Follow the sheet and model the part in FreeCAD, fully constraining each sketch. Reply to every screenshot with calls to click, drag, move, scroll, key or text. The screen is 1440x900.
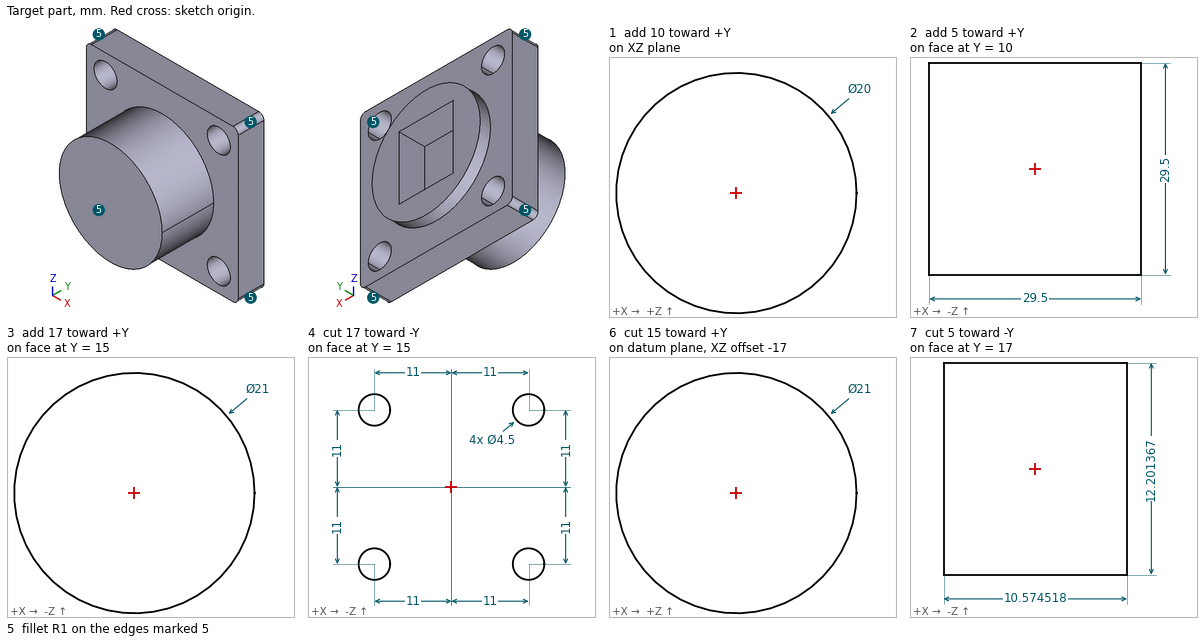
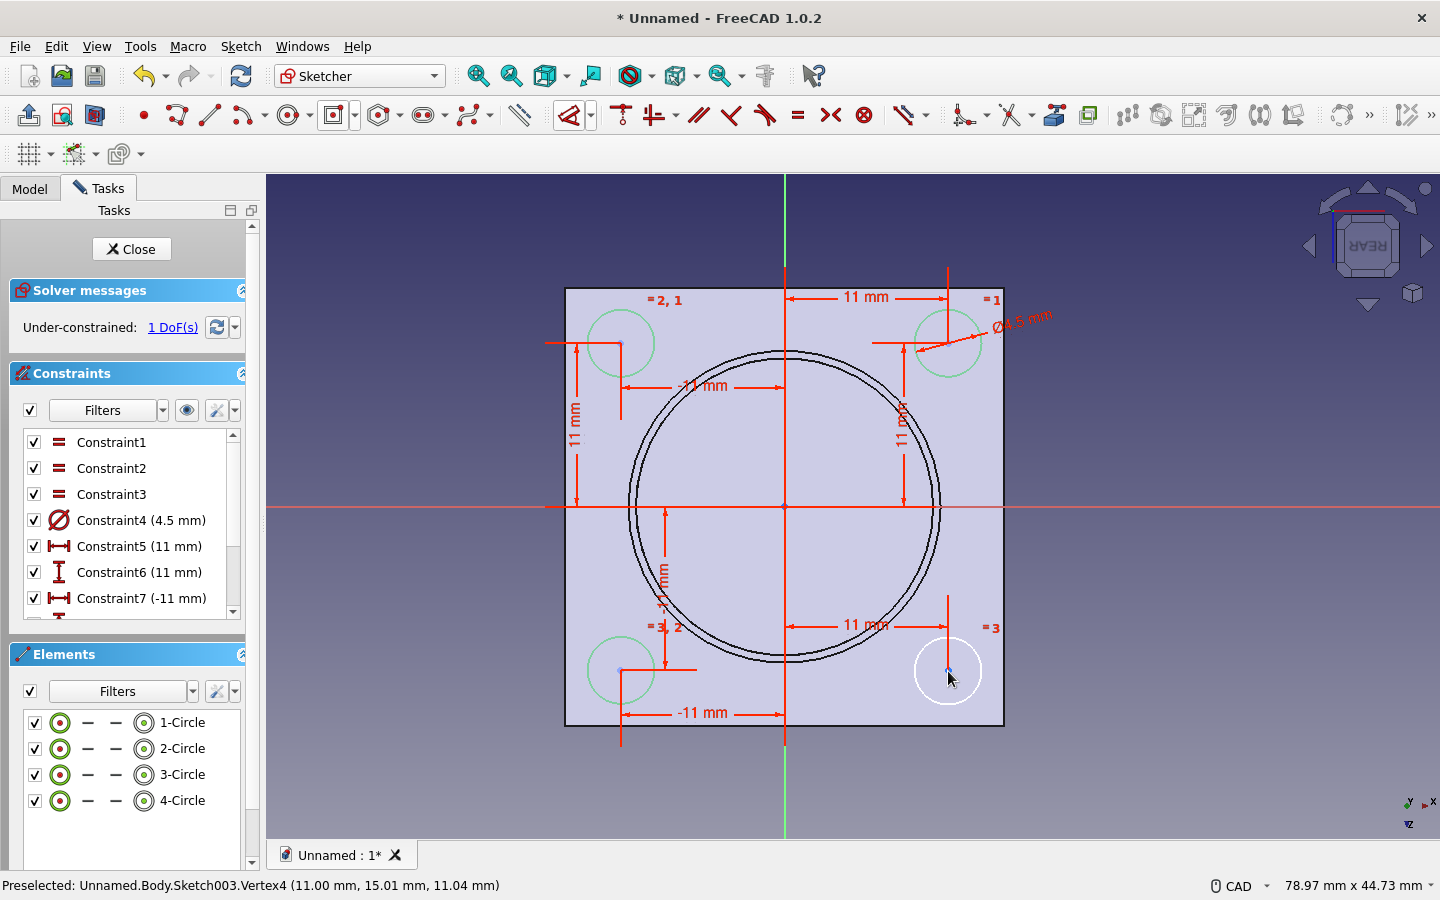
click(948, 671)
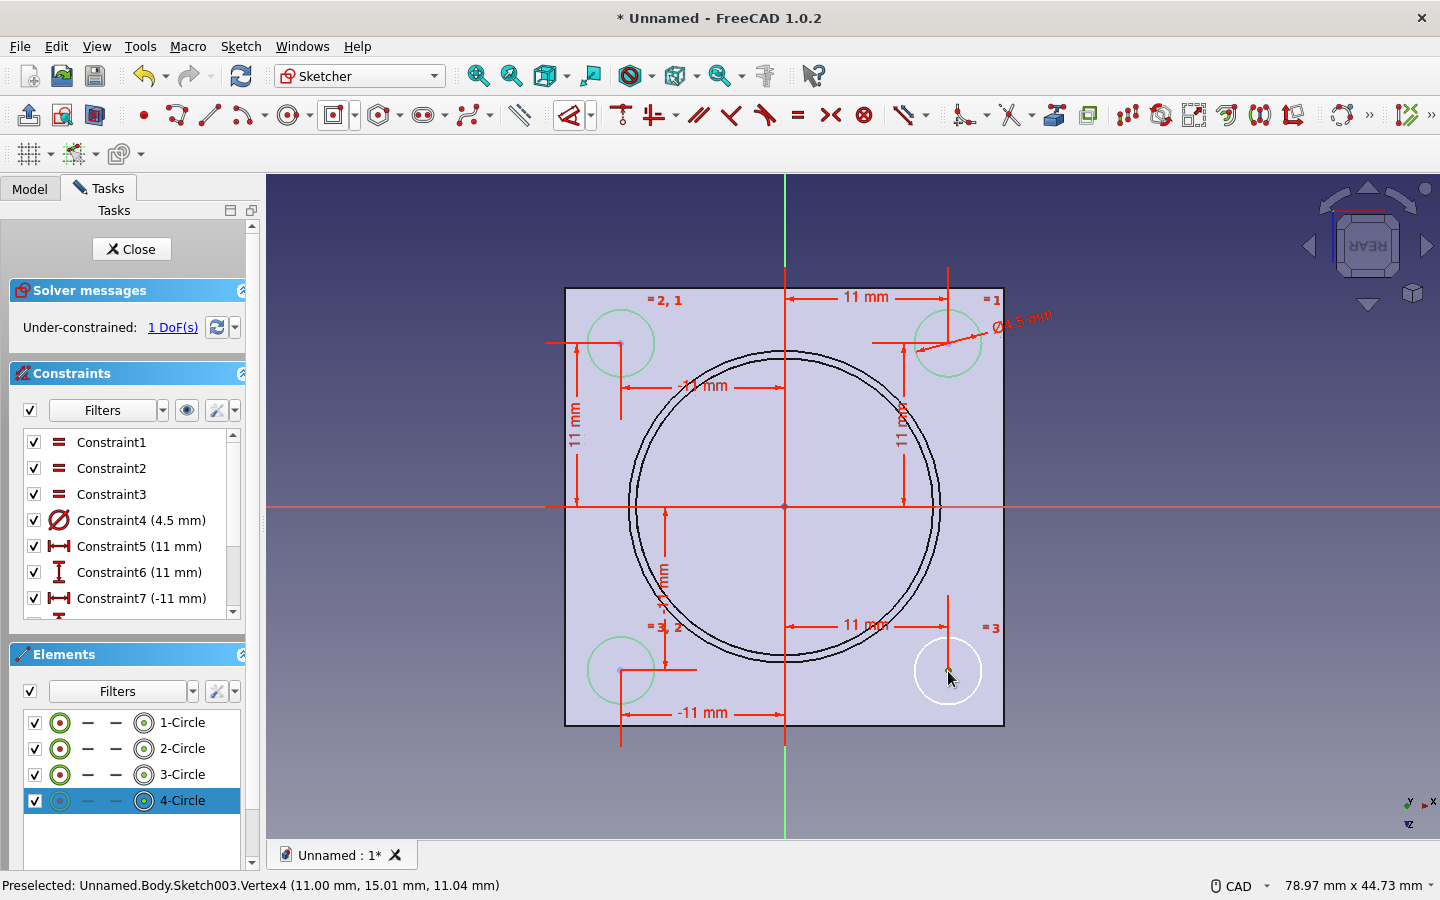
key(i)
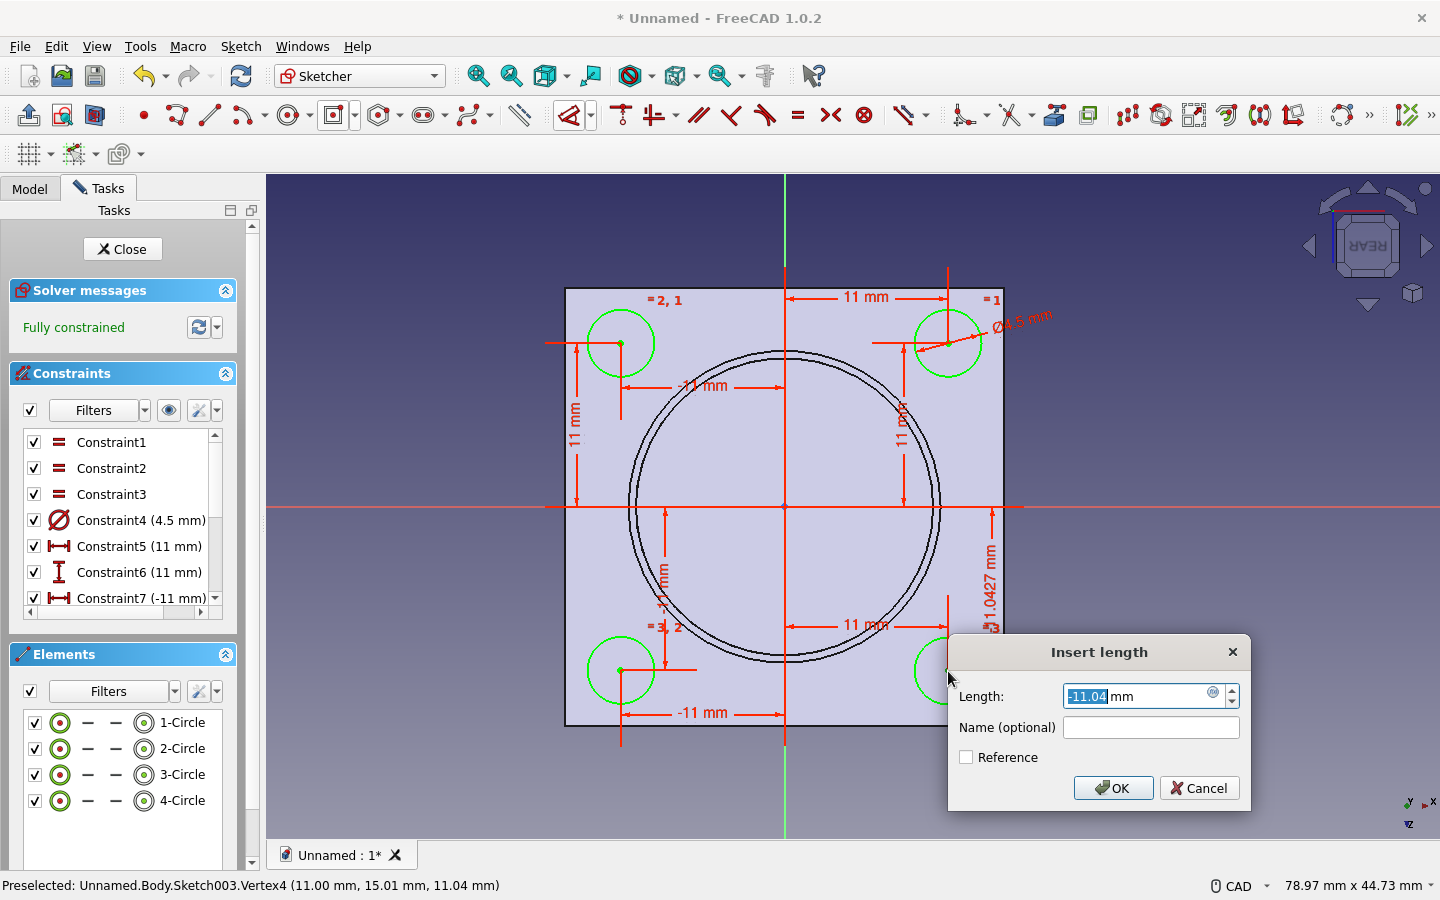
text(-11)
key(Return)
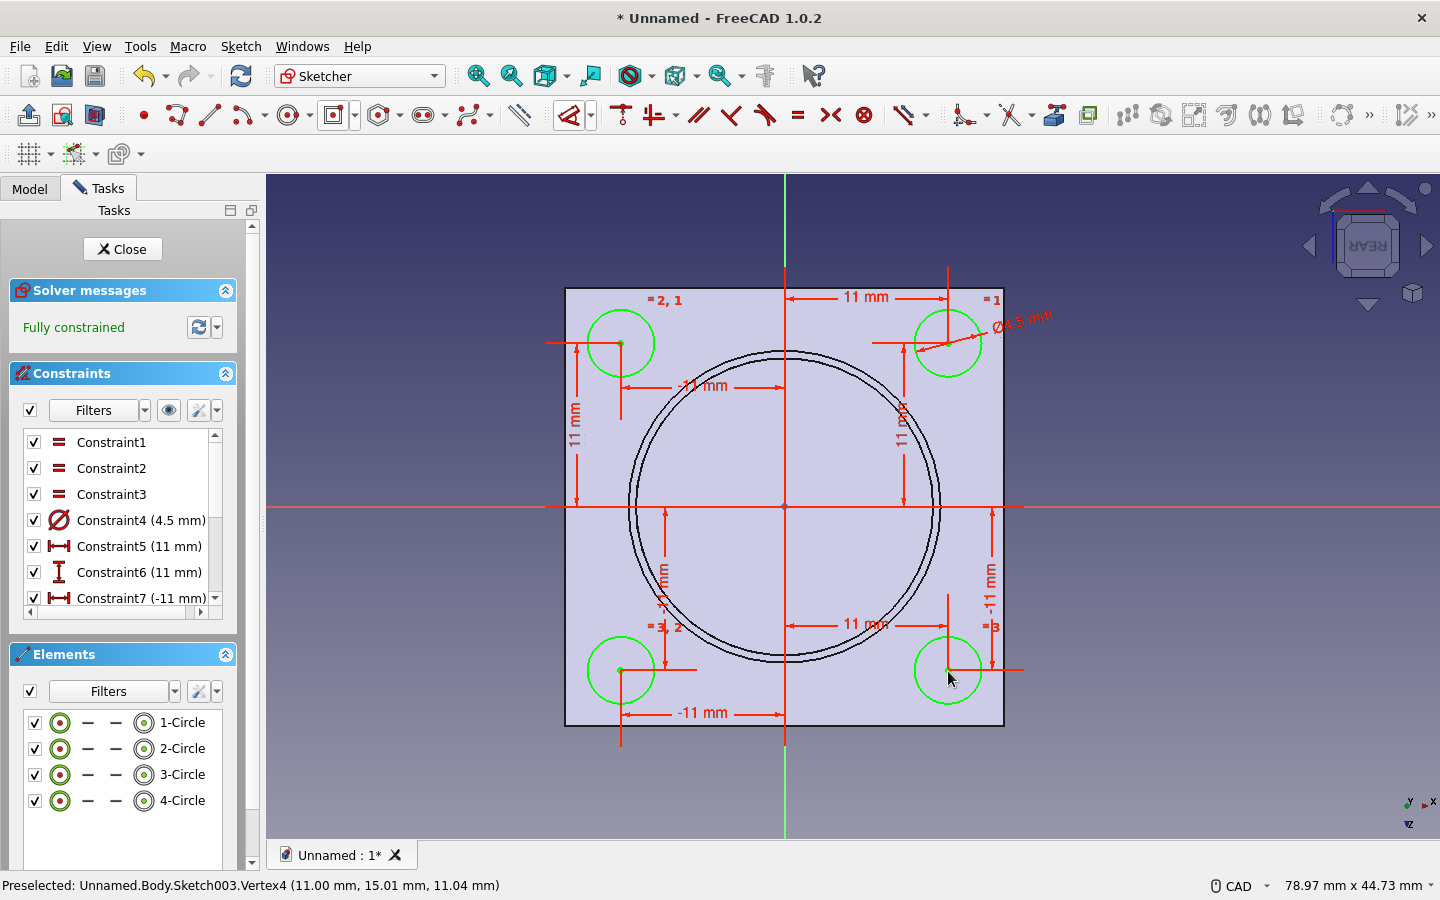
click(123, 249)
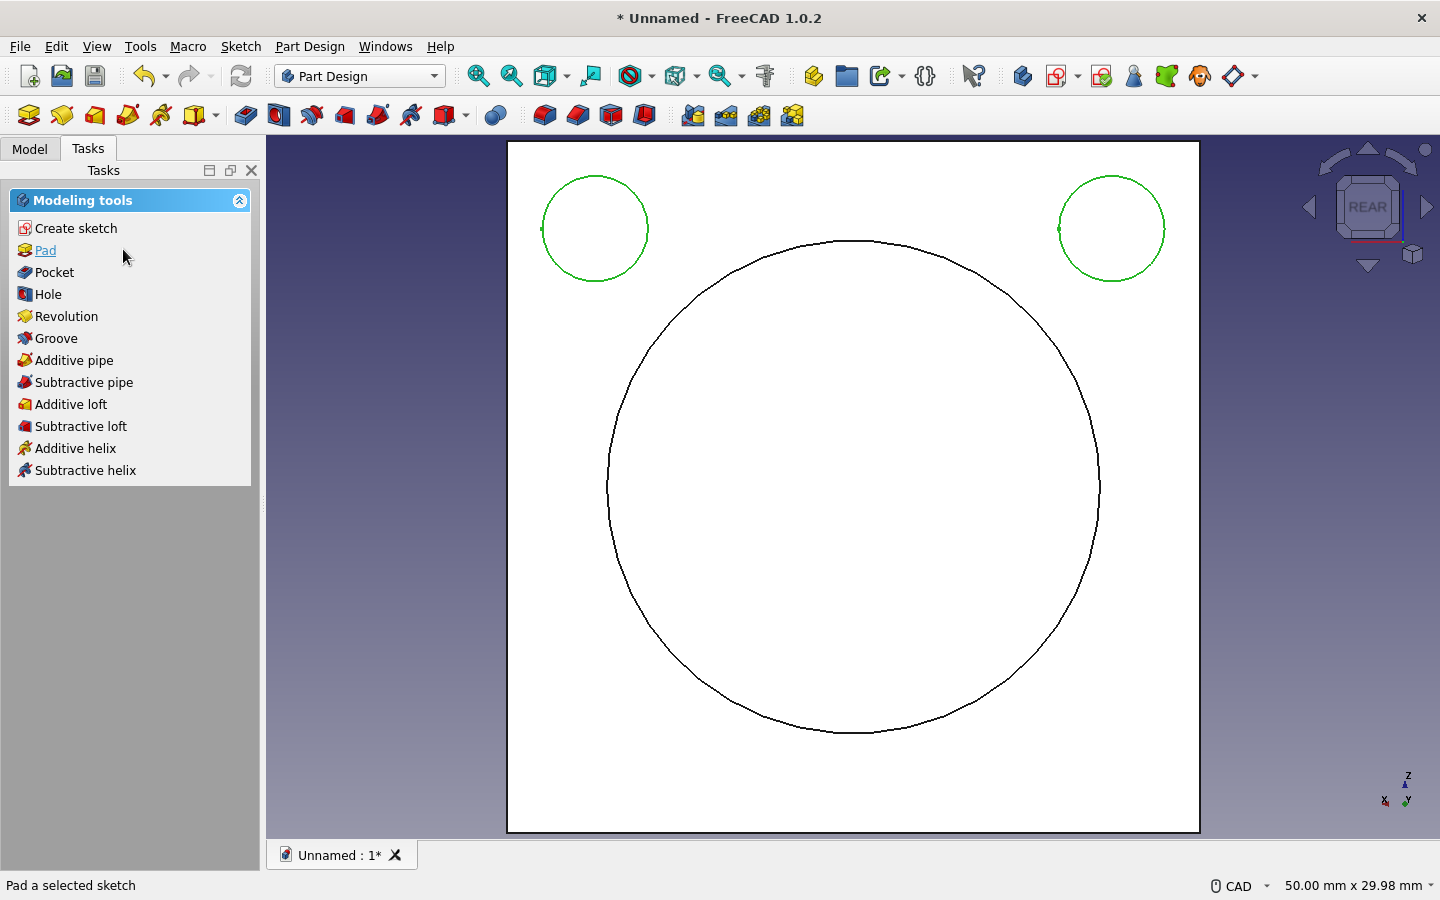
click(246, 116)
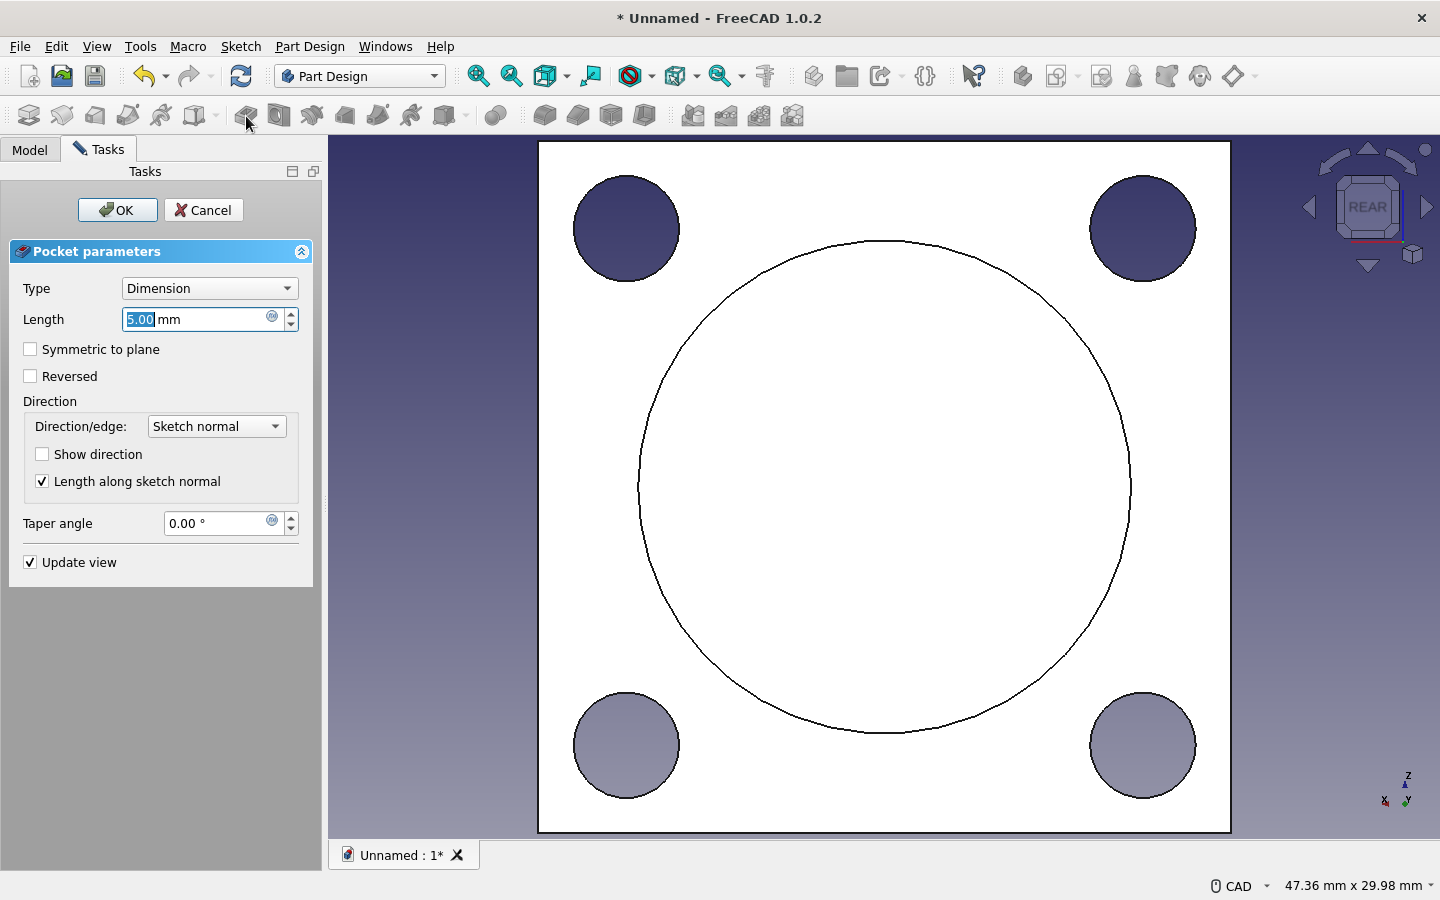
text(17)
key(Tab)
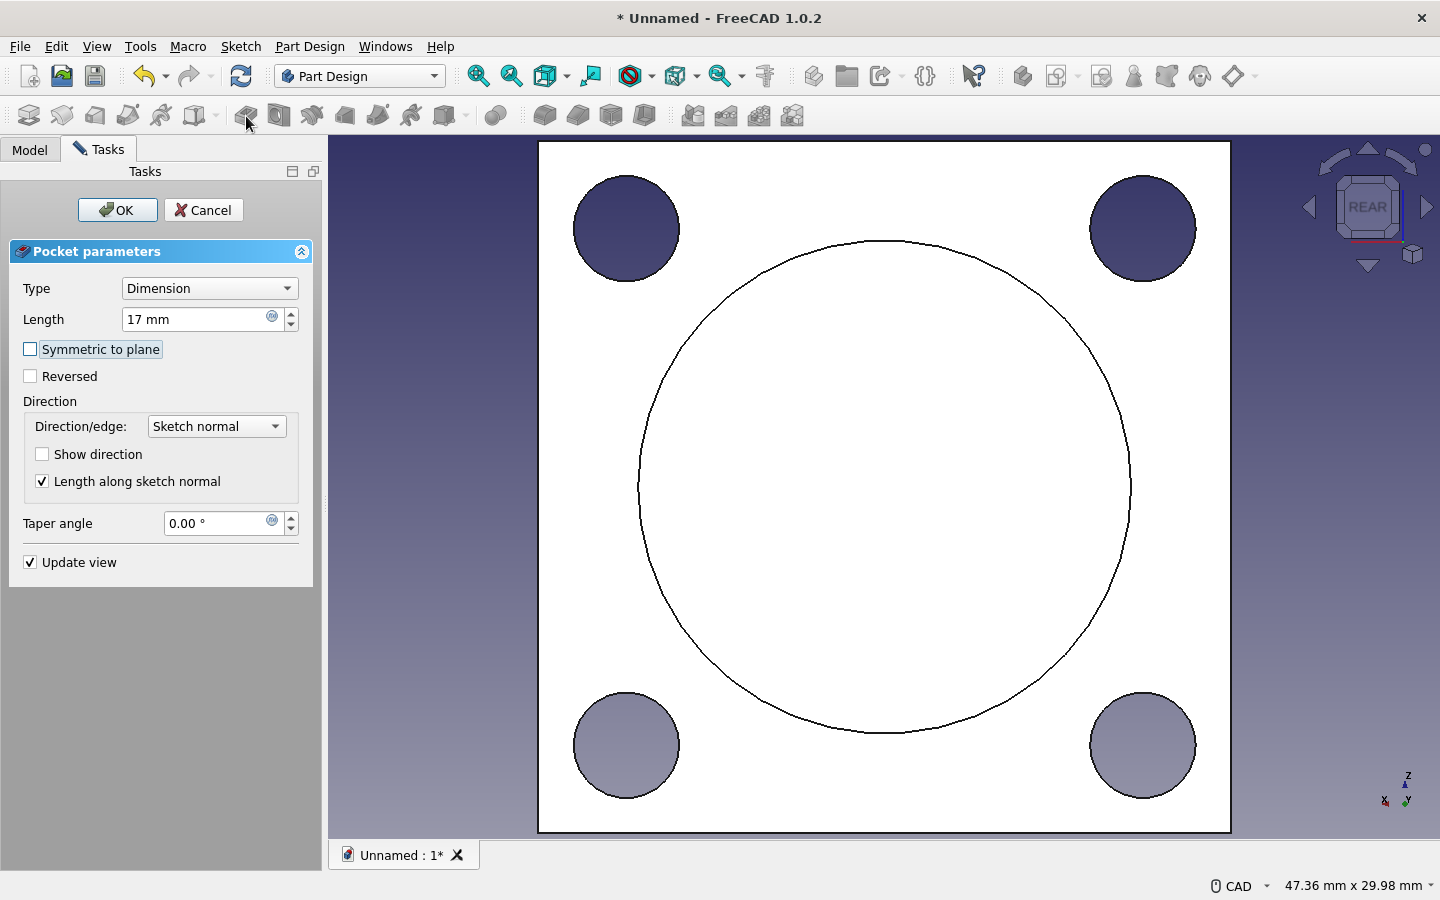
click(118, 210)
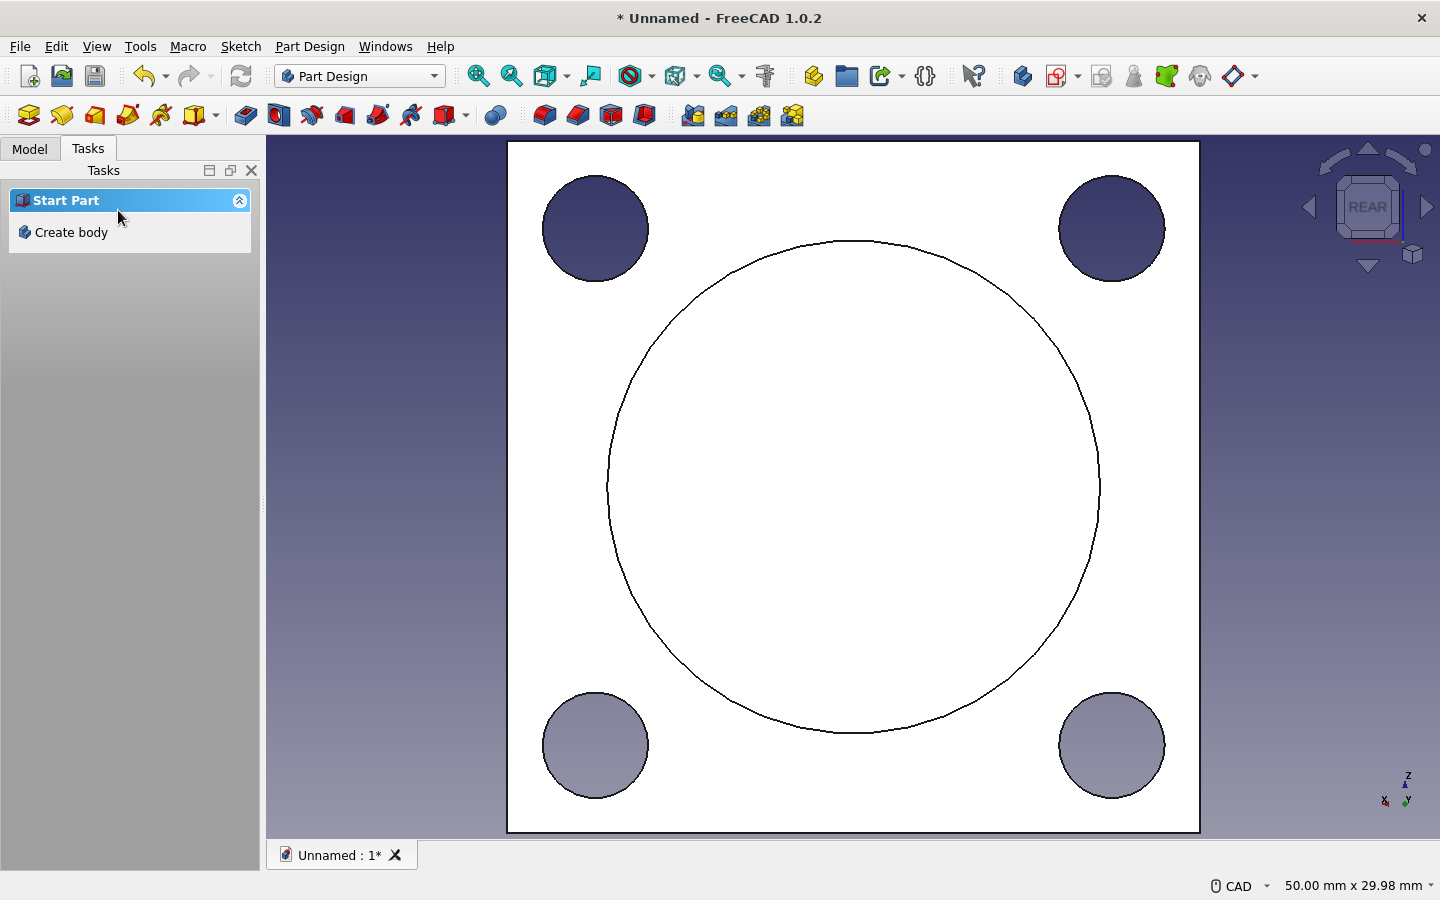
key(0)